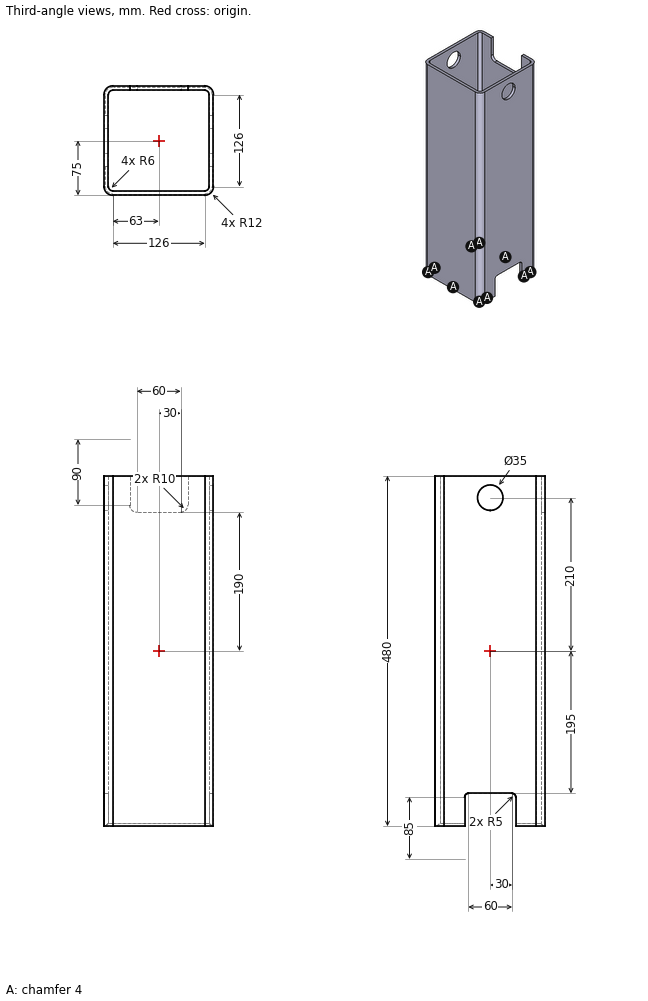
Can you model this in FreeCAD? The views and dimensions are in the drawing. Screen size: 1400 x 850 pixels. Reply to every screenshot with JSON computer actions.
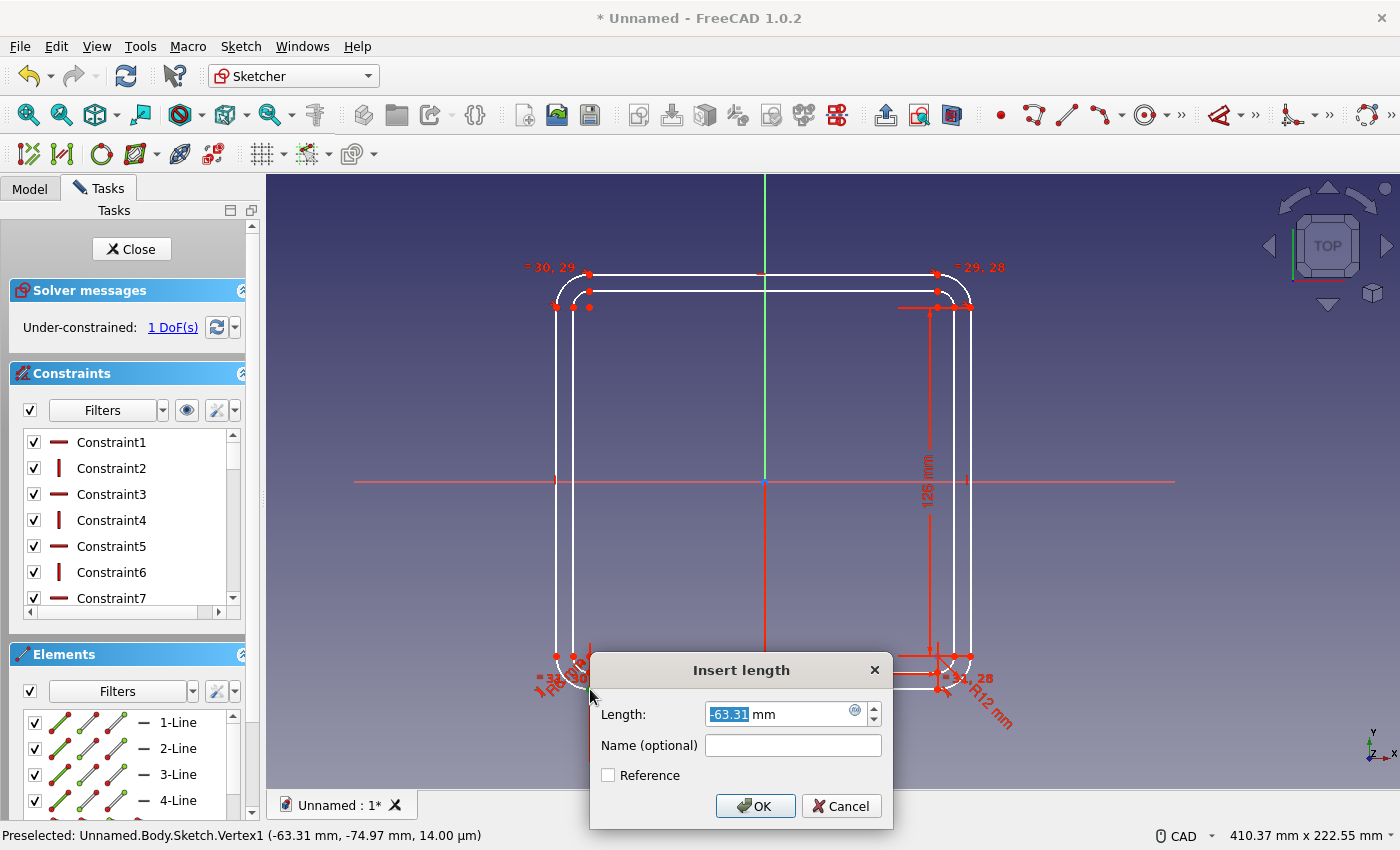
{"action": "type", "text": "-63"}
{"action": "key", "text": "Return"}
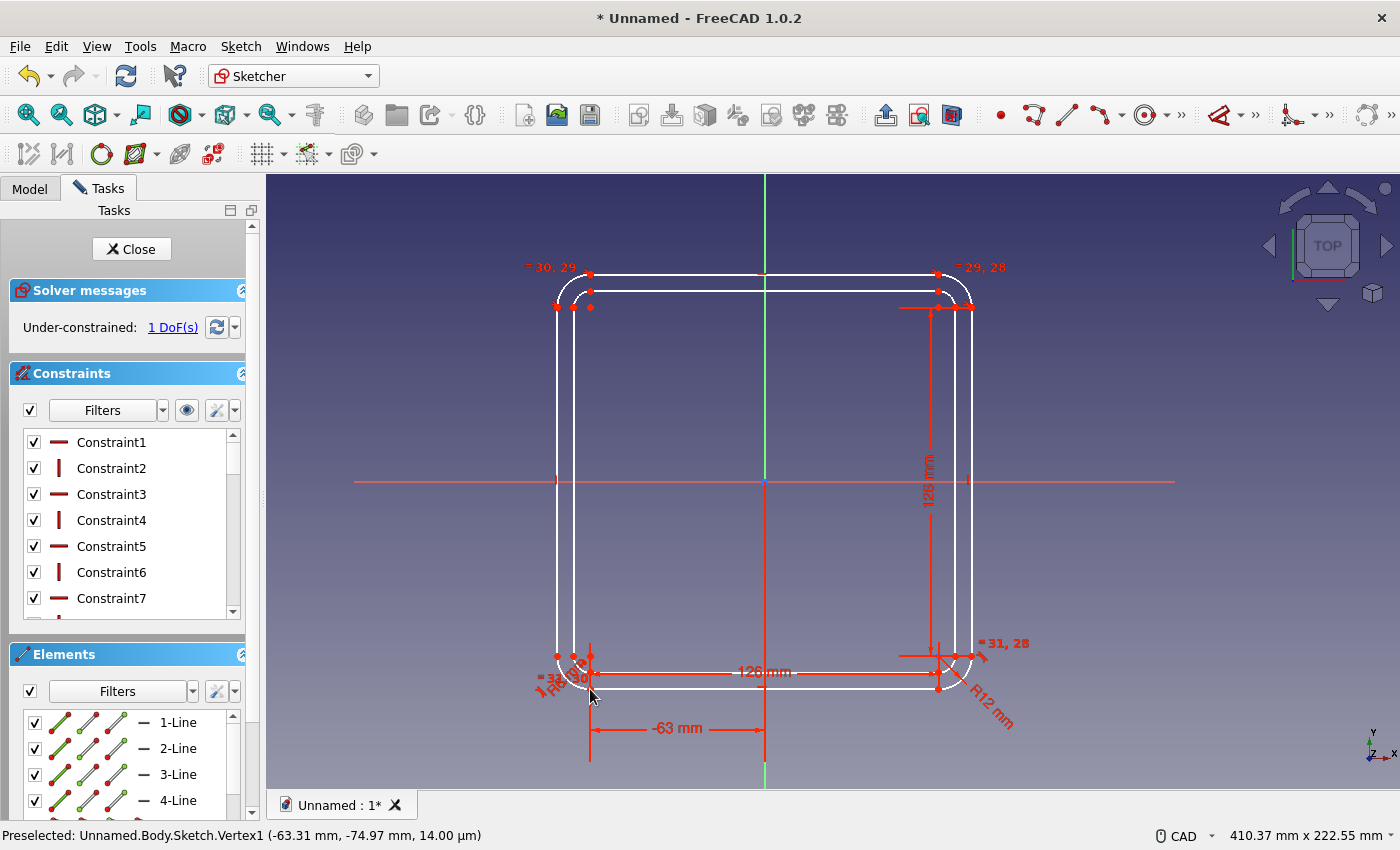
{"action": "left_click", "coordinate": [590, 689]}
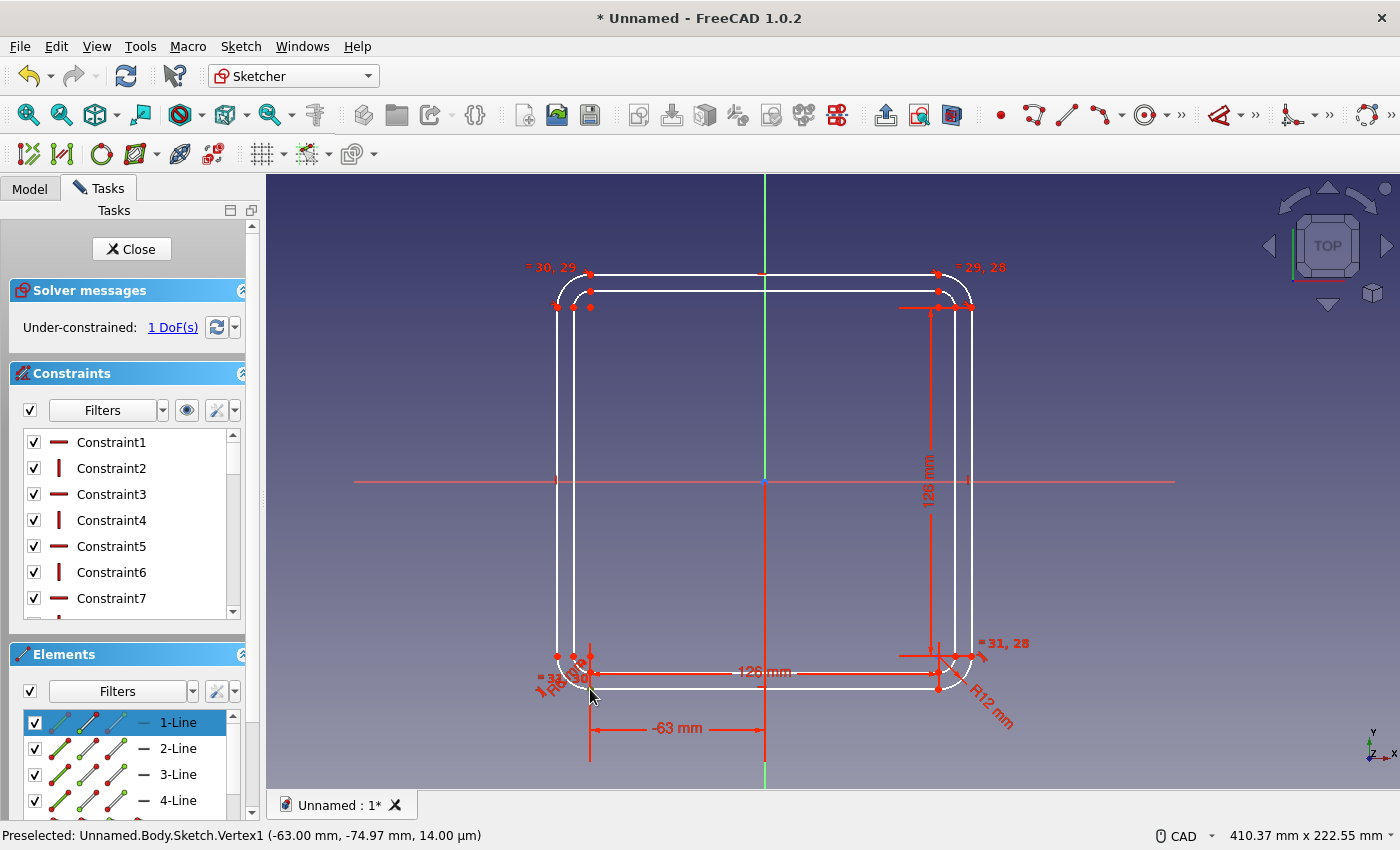
{"action": "key", "text": "i"}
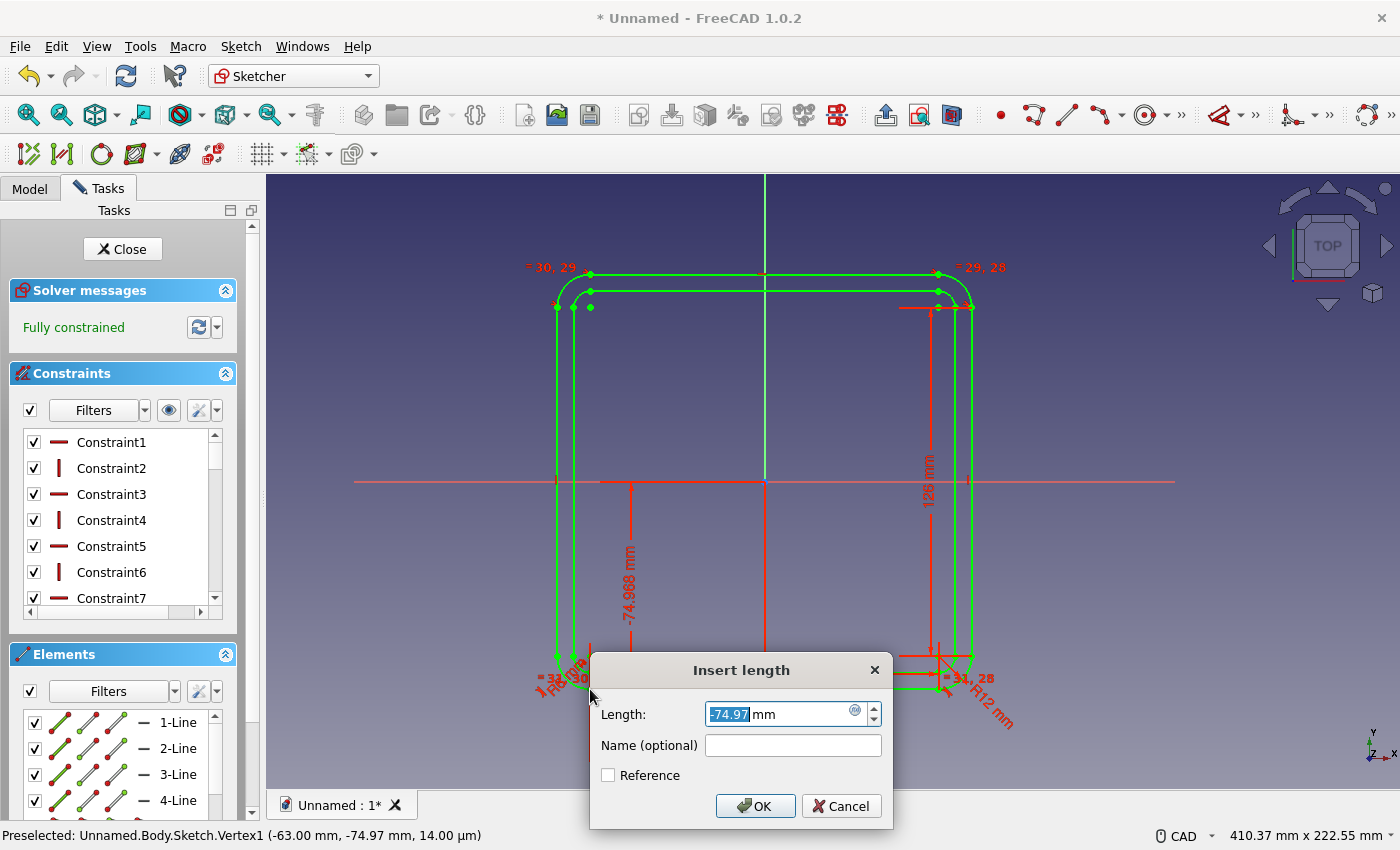
{"action": "type", "text": "-75"}
{"action": "key", "text": "Return"}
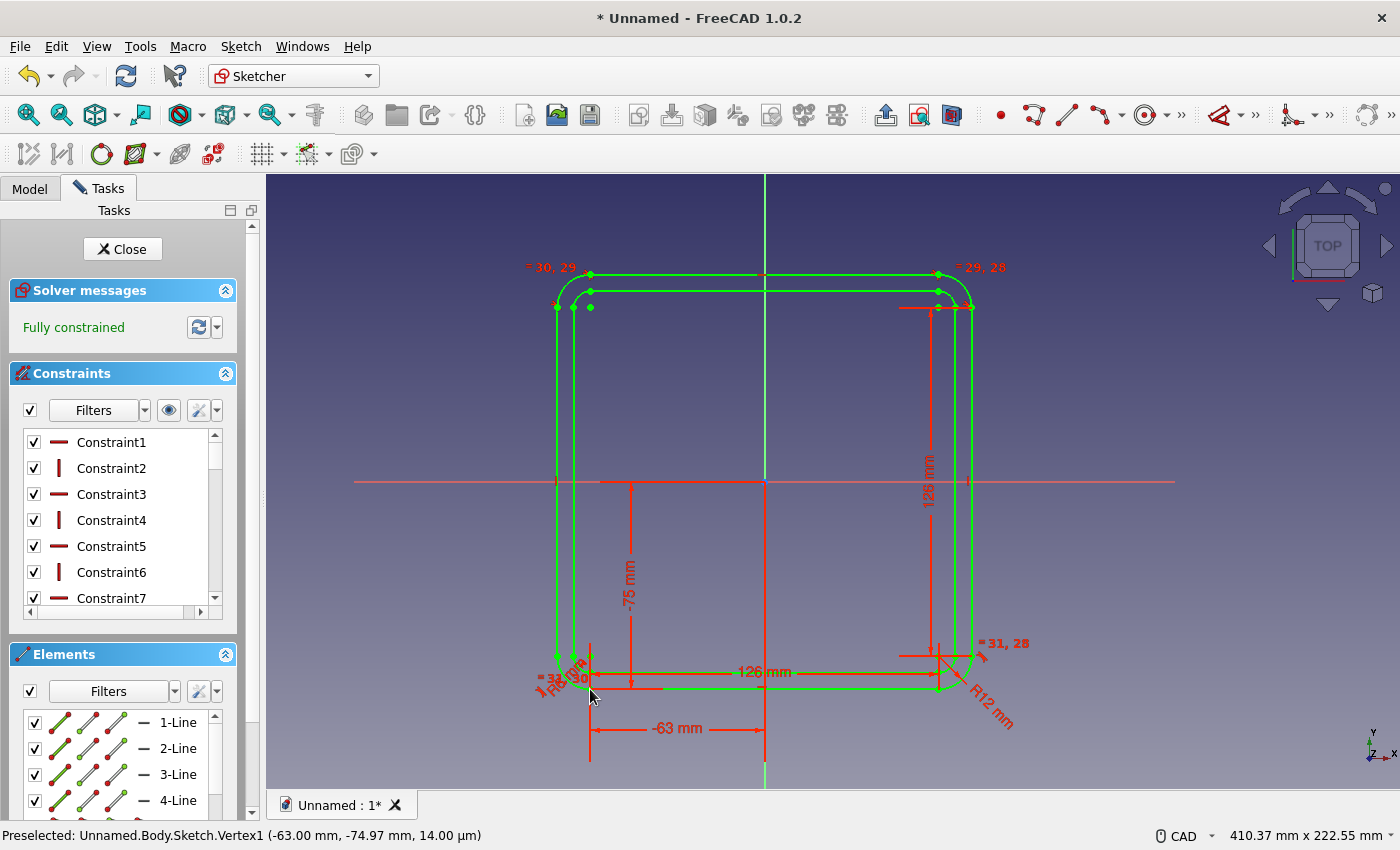
{"action": "left_click", "coordinate": [123, 249]}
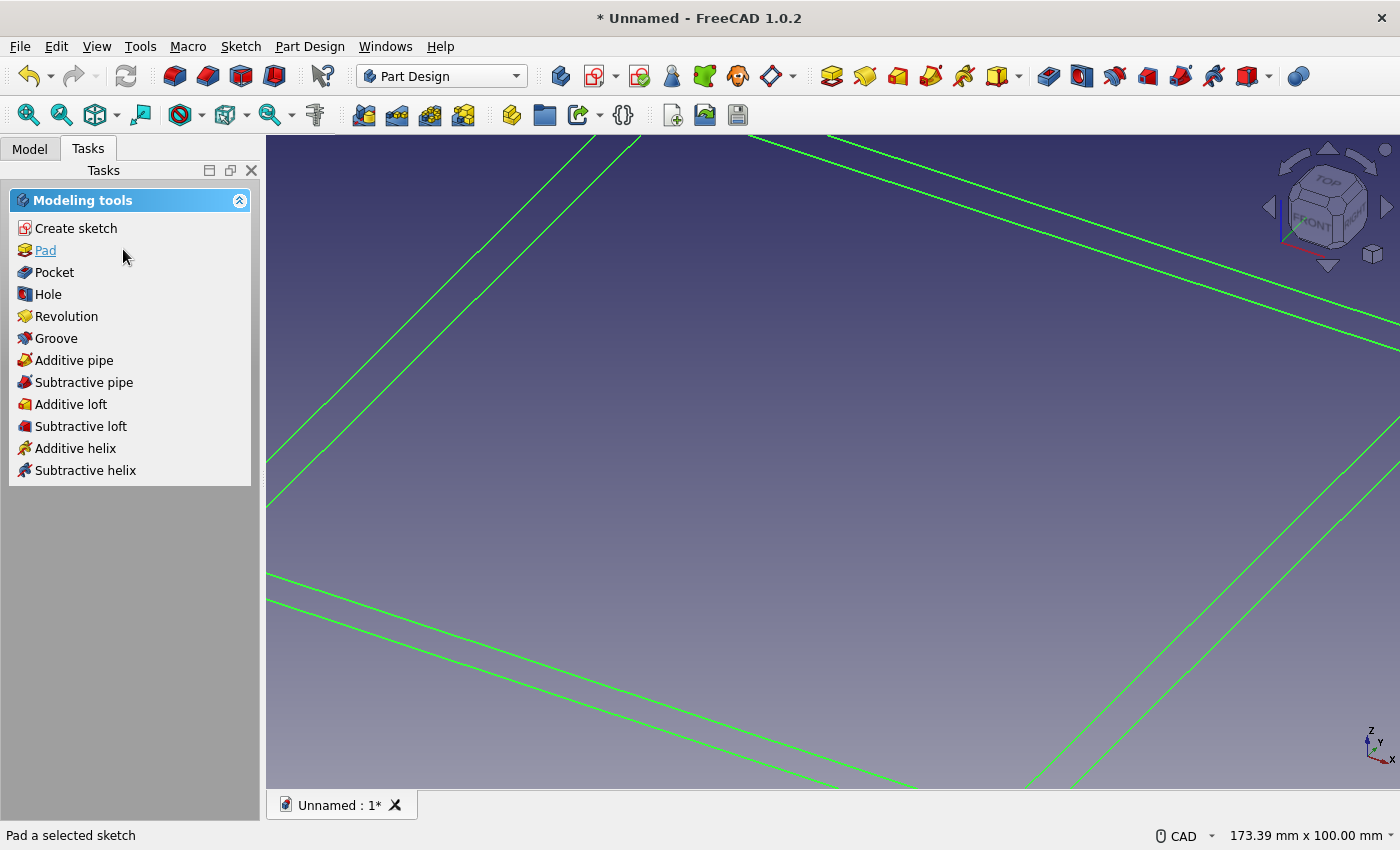
{"action": "left_click", "coordinate": [832, 76]}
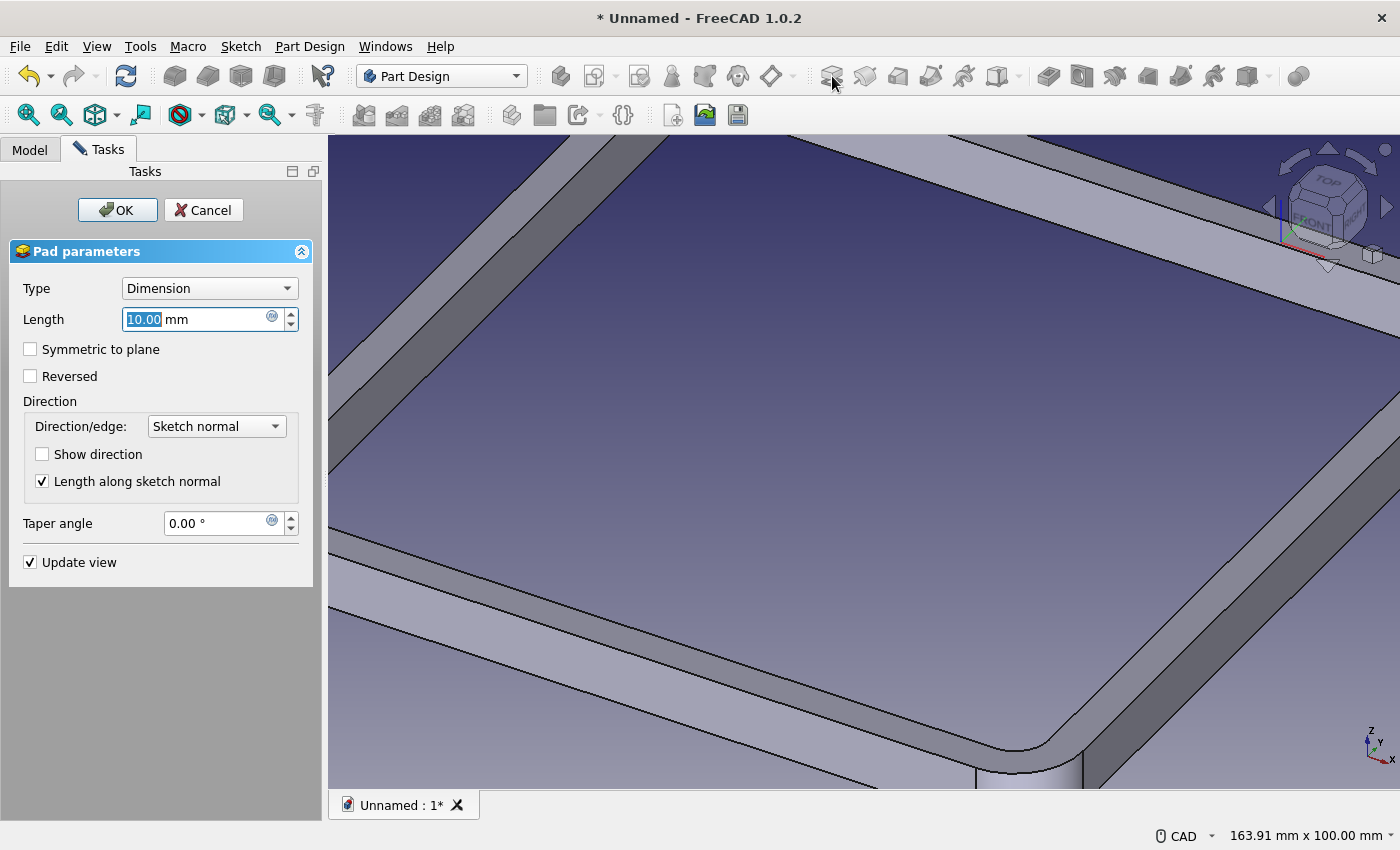
{"action": "type", "text": "480"}
{"action": "key", "text": "Tab"}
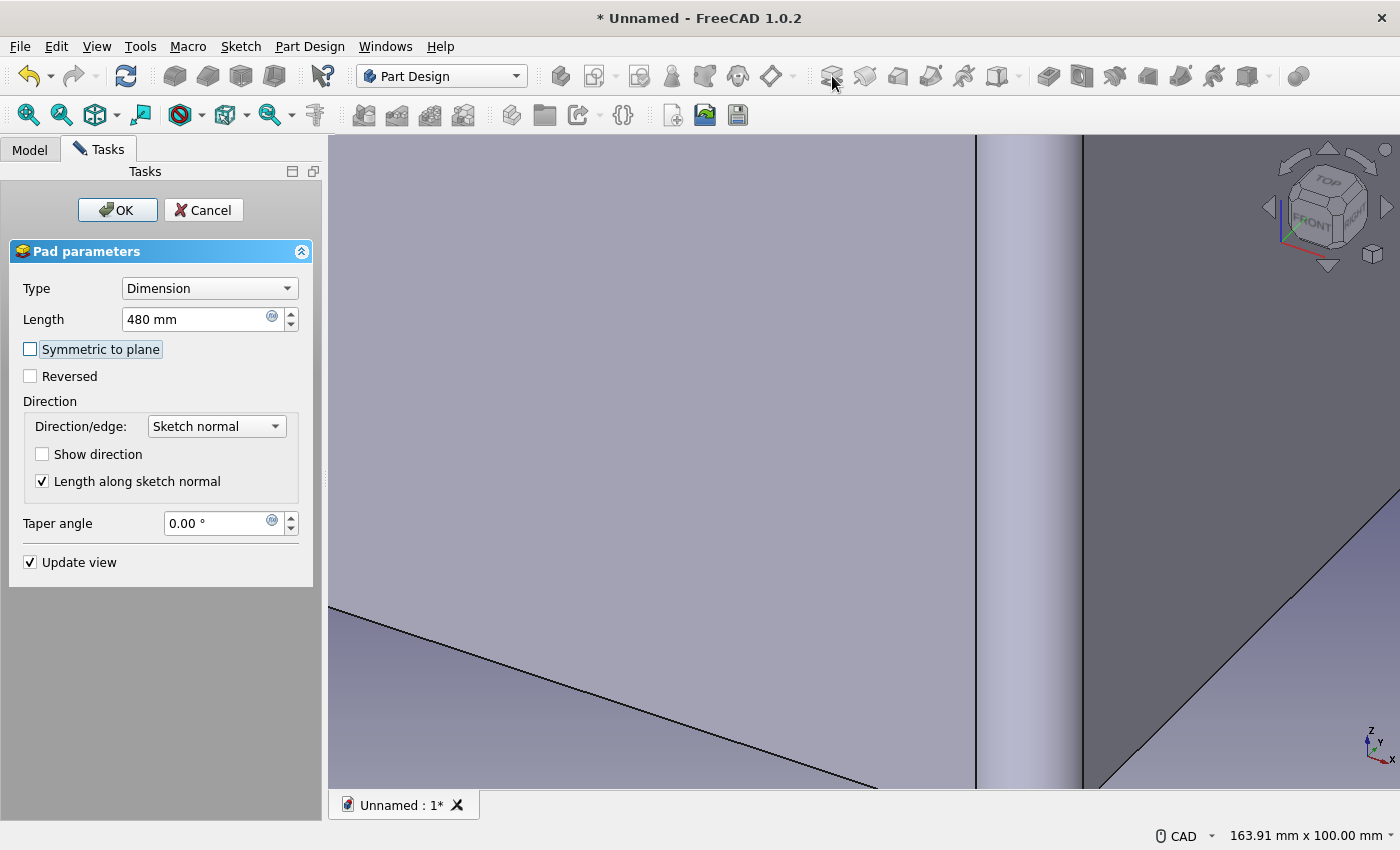
{"action": "left_click", "coordinate": [31, 349]}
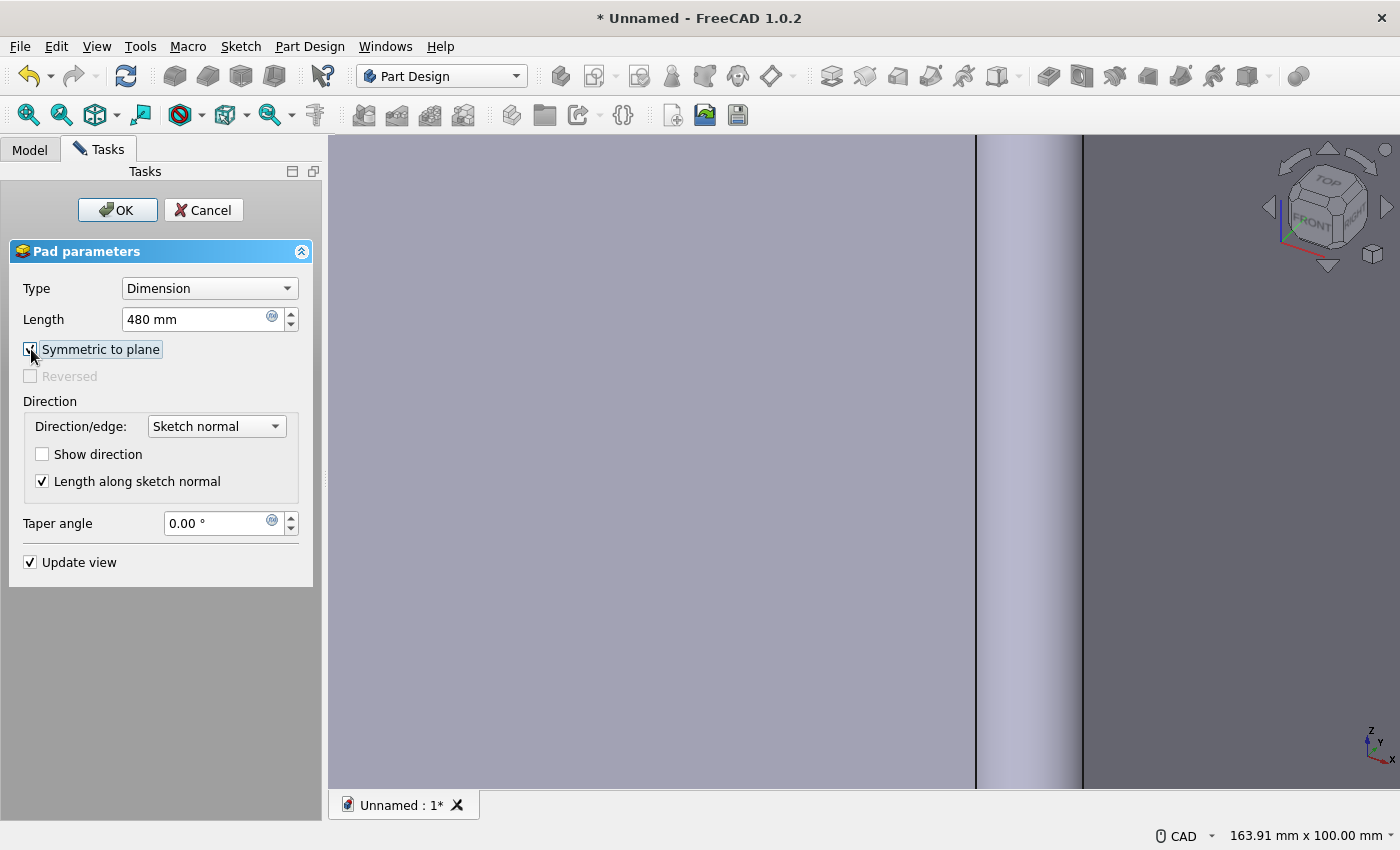
{"action": "left_click", "coordinate": [118, 210]}